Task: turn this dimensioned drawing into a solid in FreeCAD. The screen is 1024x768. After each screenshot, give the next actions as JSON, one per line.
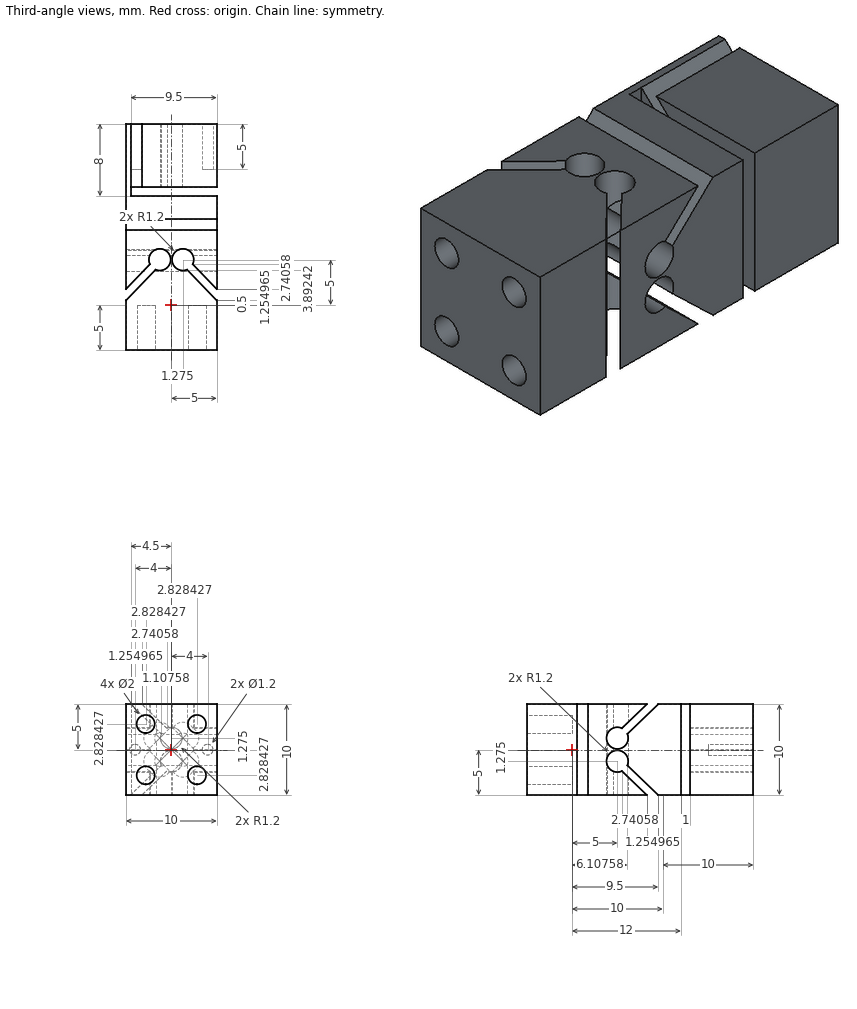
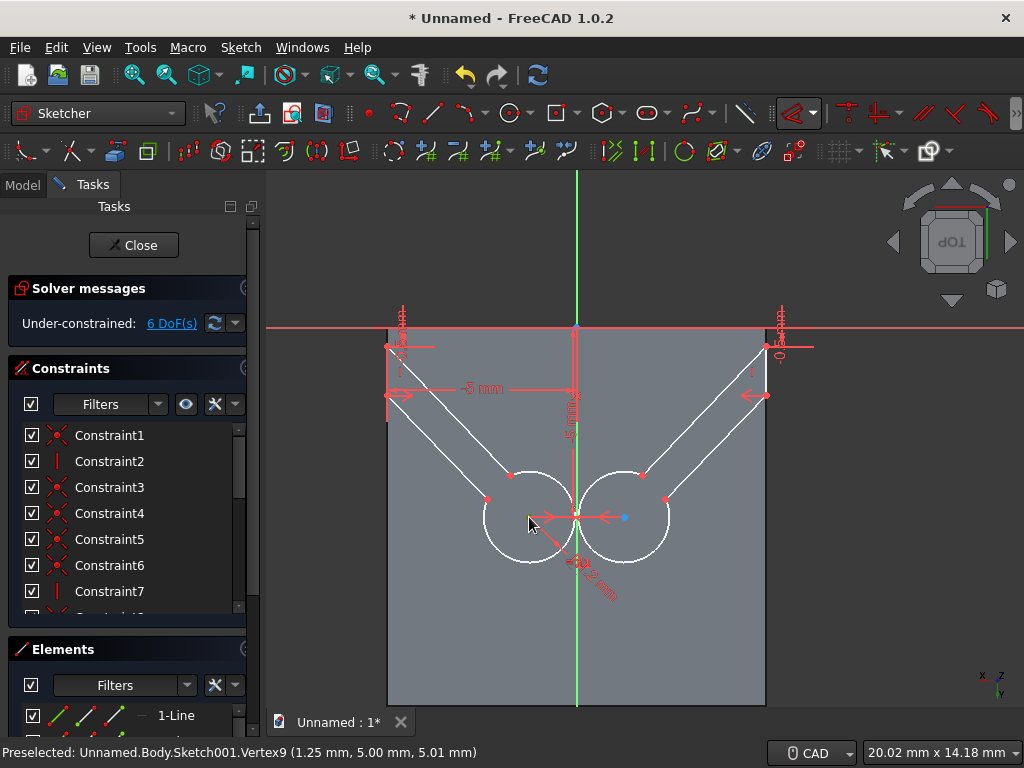
{"action": "left_click", "coordinate": [816, 114]}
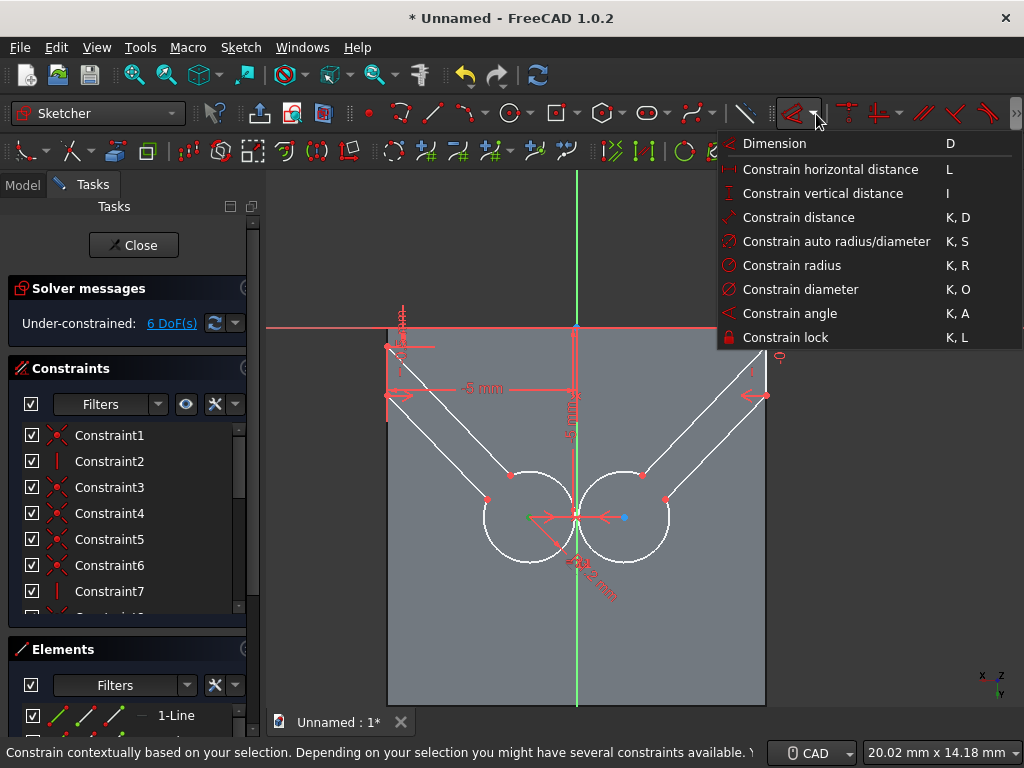
{"action": "left_click", "coordinate": [870, 169]}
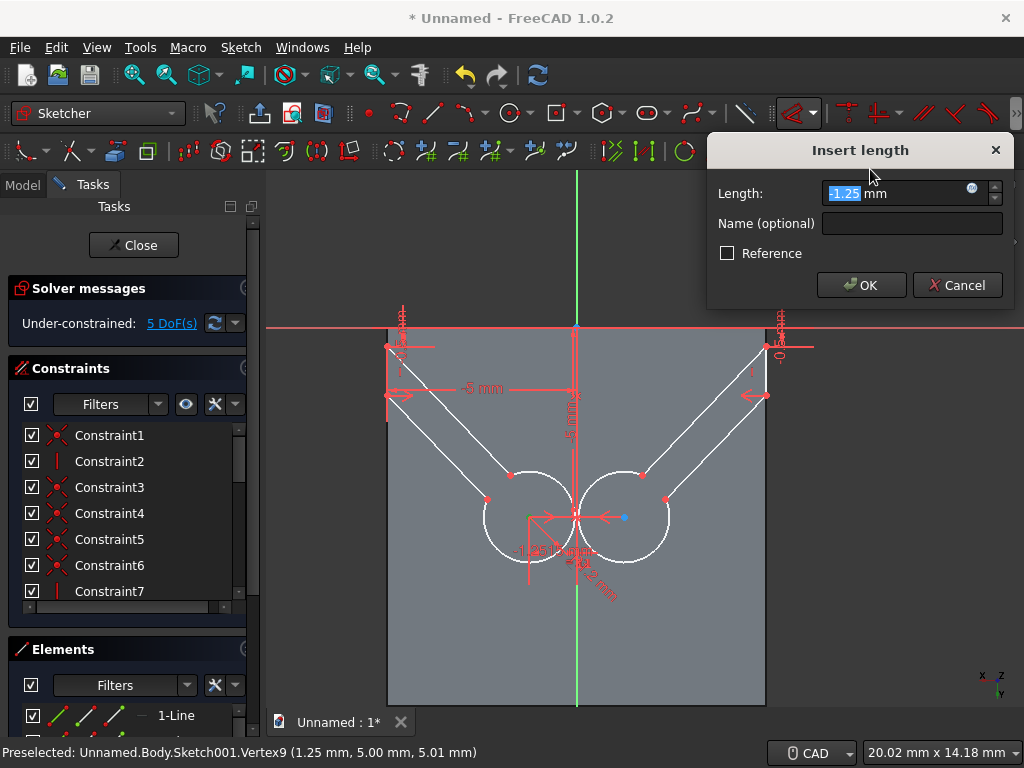
{"action": "type", "text": "-1.275"}
{"action": "key", "text": "Return"}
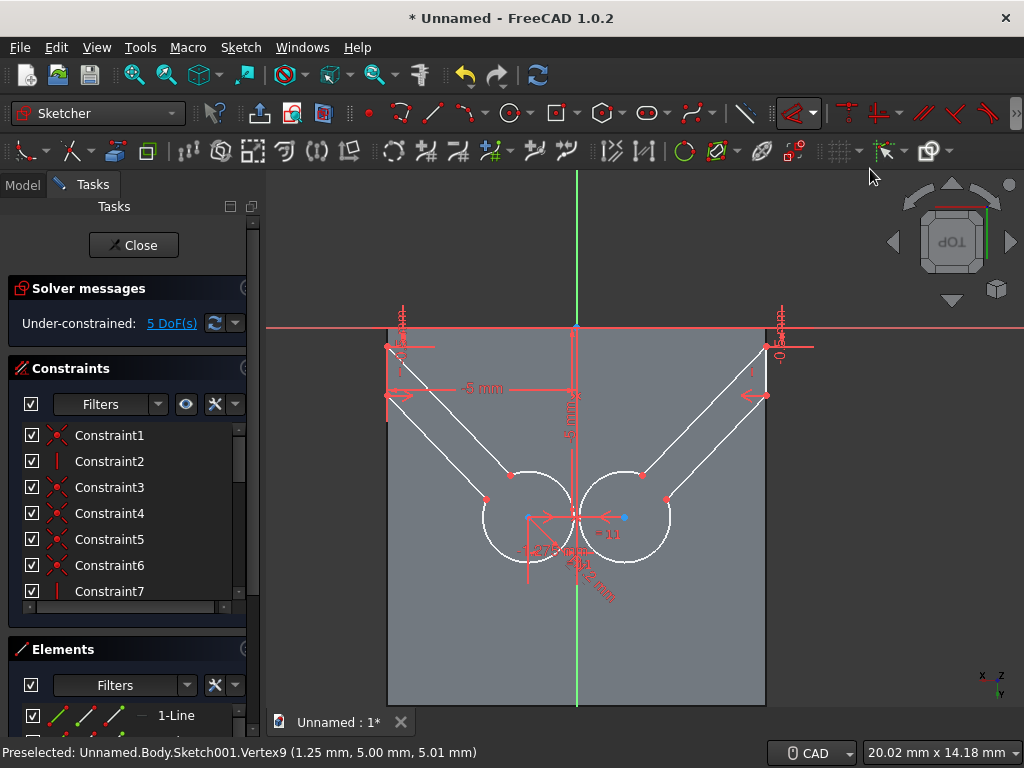
{"action": "scroll", "coordinate": [387, 361], "scroll_direction": "up", "scroll_amount": 2}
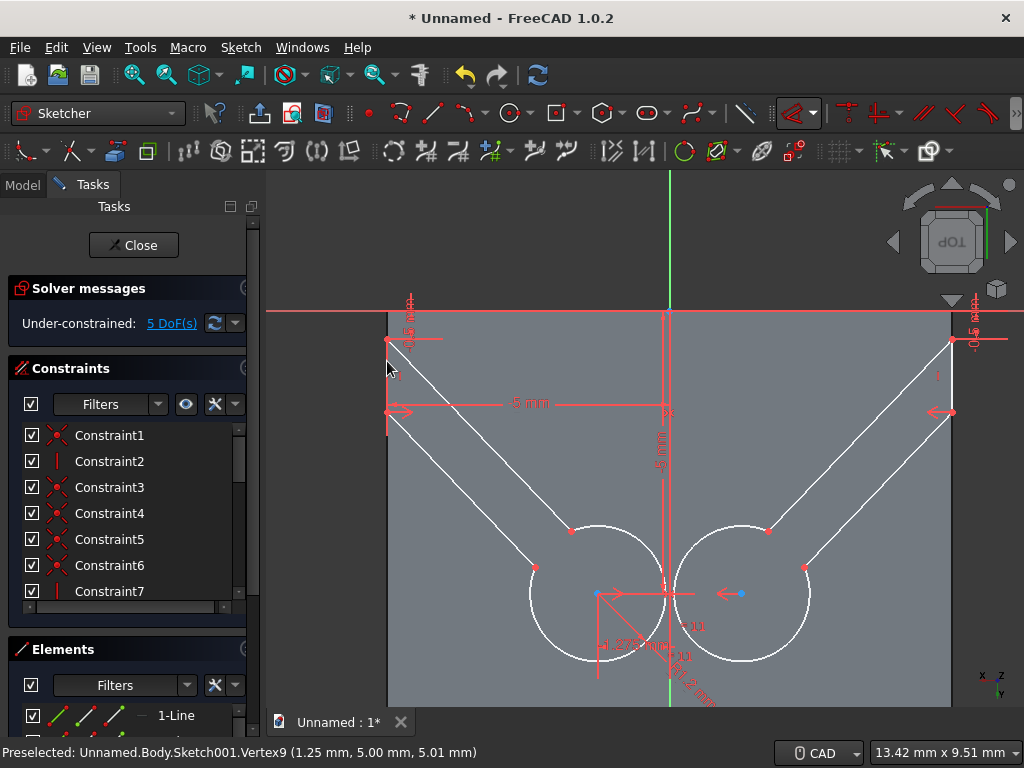
{"action": "left_click", "coordinate": [387, 361]}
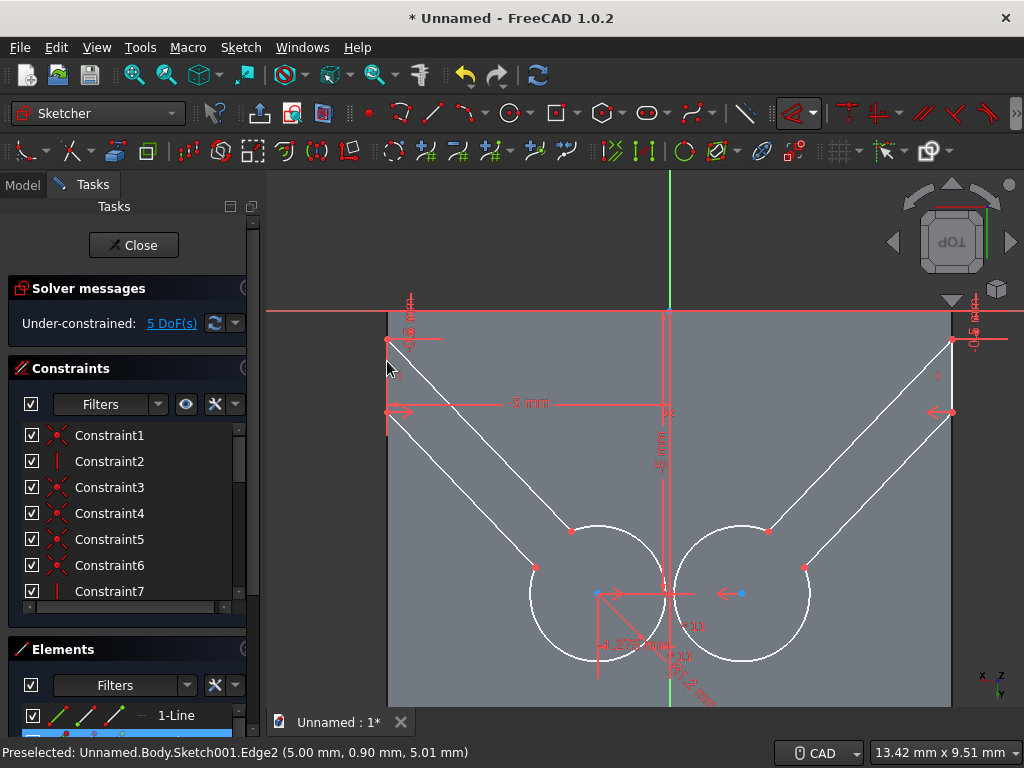
{"action": "left_click", "coordinate": [816, 114]}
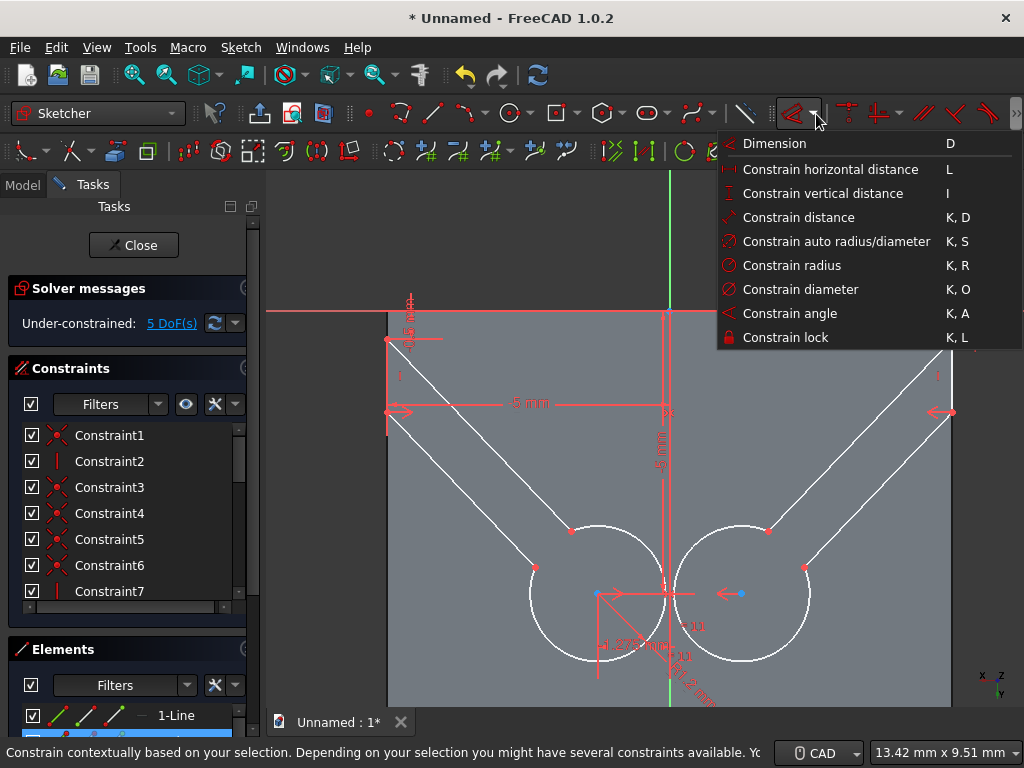
{"action": "left_click", "coordinate": [870, 193]}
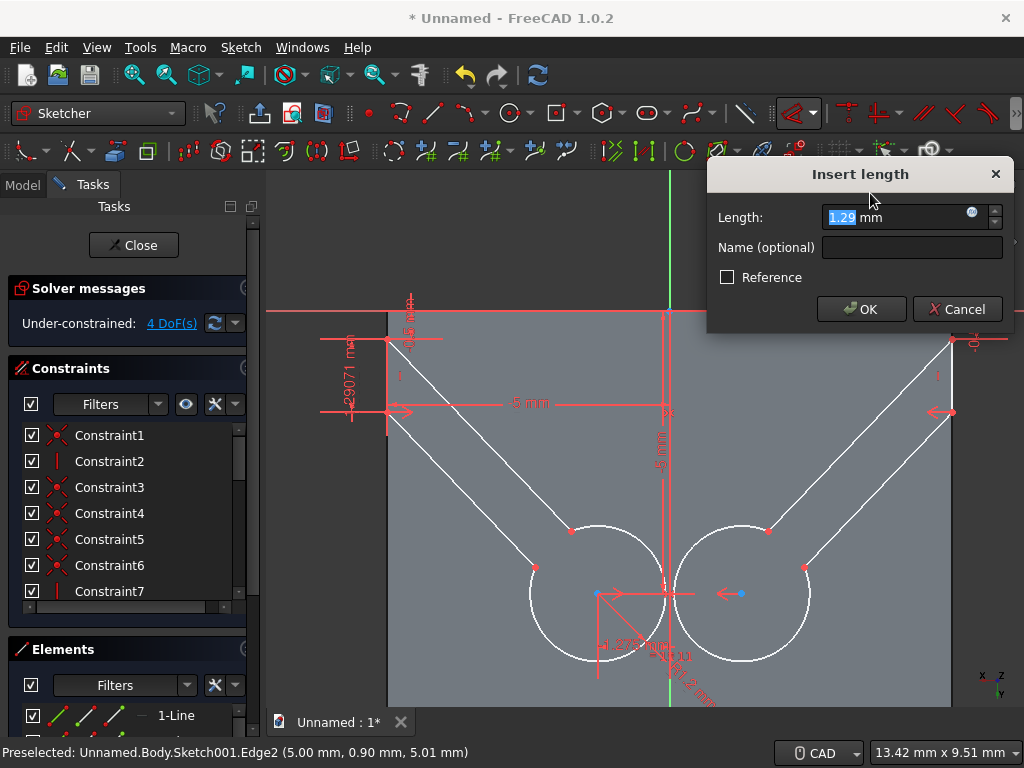
{"action": "type", "text": "1.254965"}
{"action": "key", "text": "Return"}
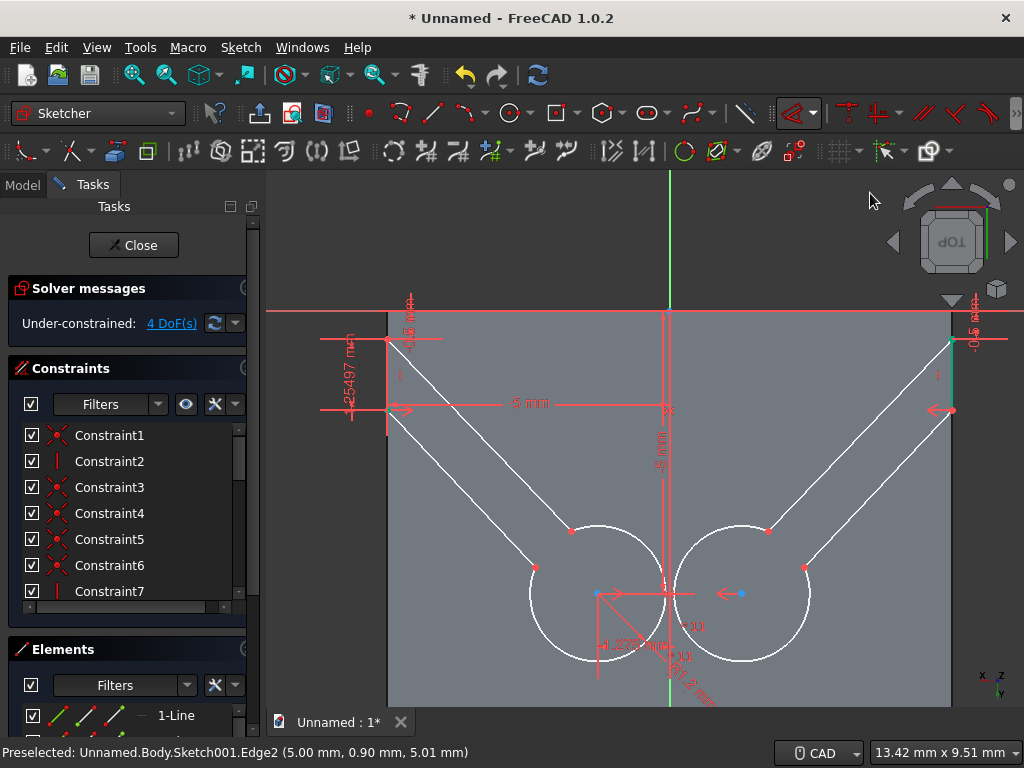
{"action": "left_click", "coordinate": [572, 531]}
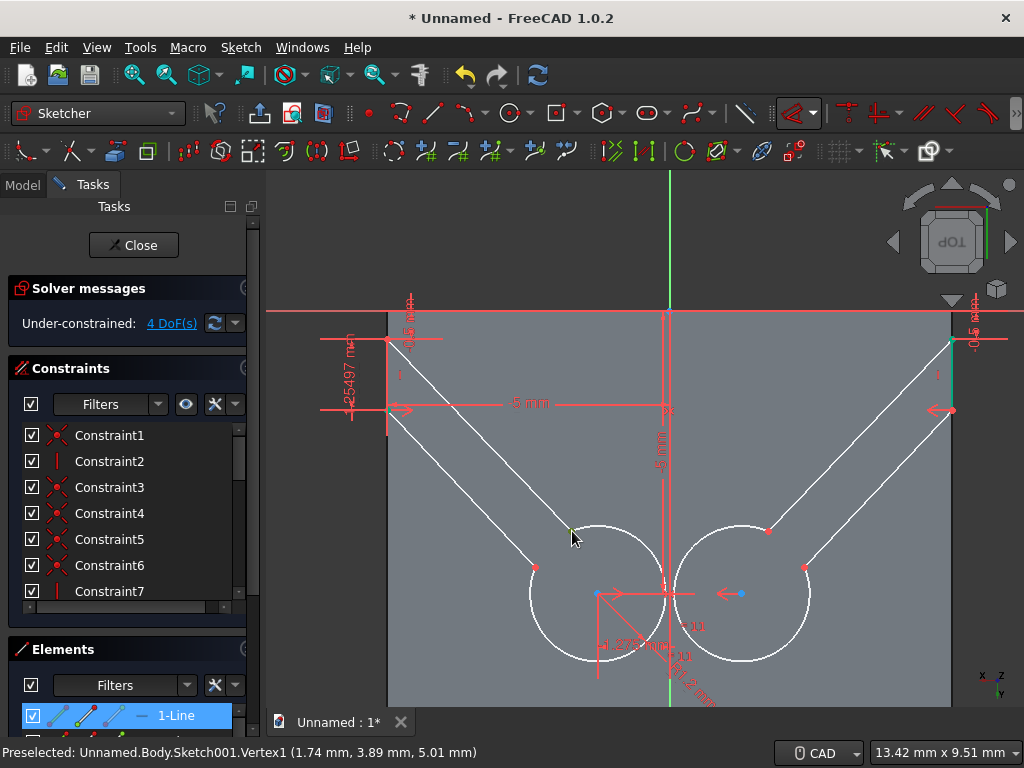
{"action": "key", "text": "i"}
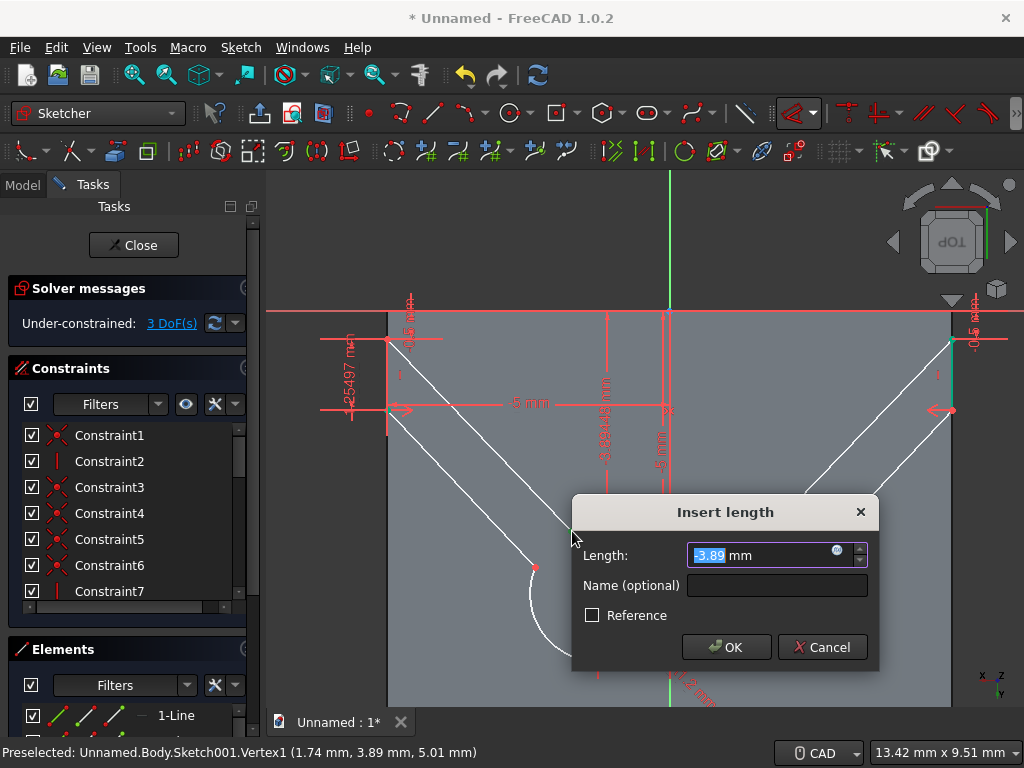
{"action": "type", "text": "-3.89242"}
{"action": "key", "text": "Return"}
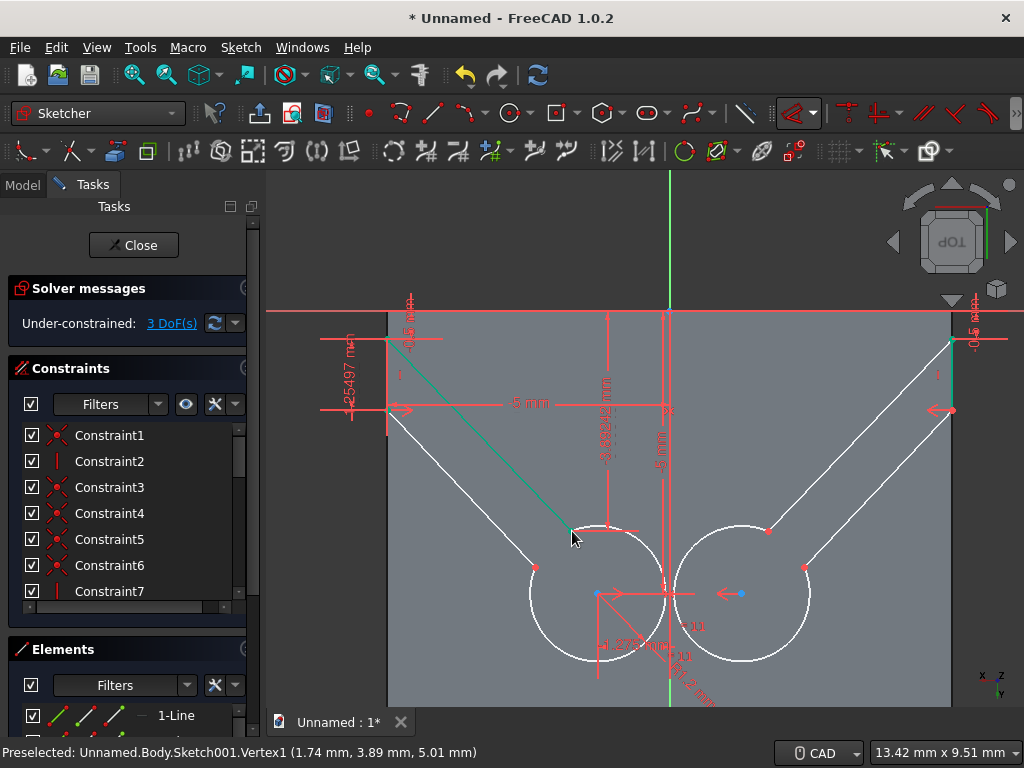
{"action": "left_click", "coordinate": [768, 531]}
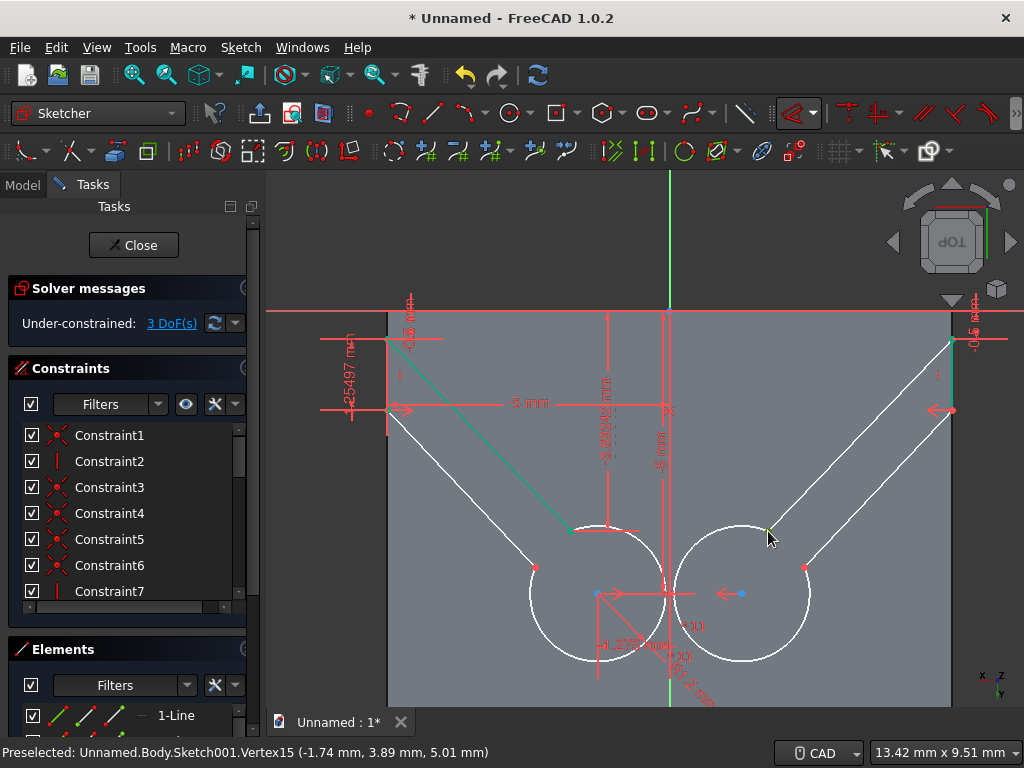
{"action": "key", "text": "i"}